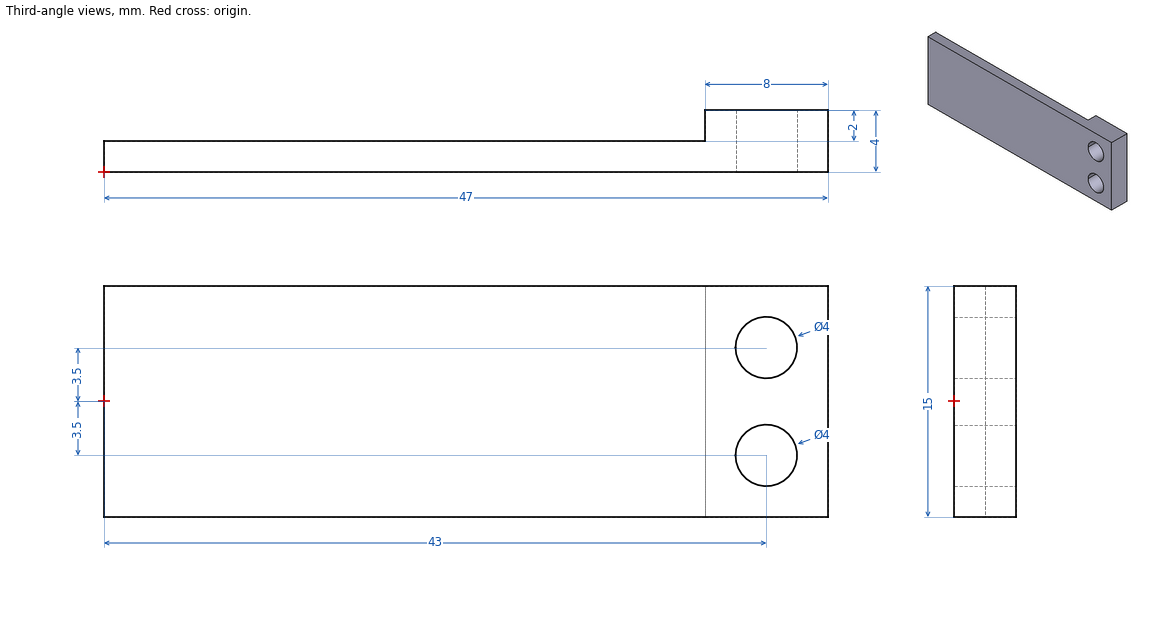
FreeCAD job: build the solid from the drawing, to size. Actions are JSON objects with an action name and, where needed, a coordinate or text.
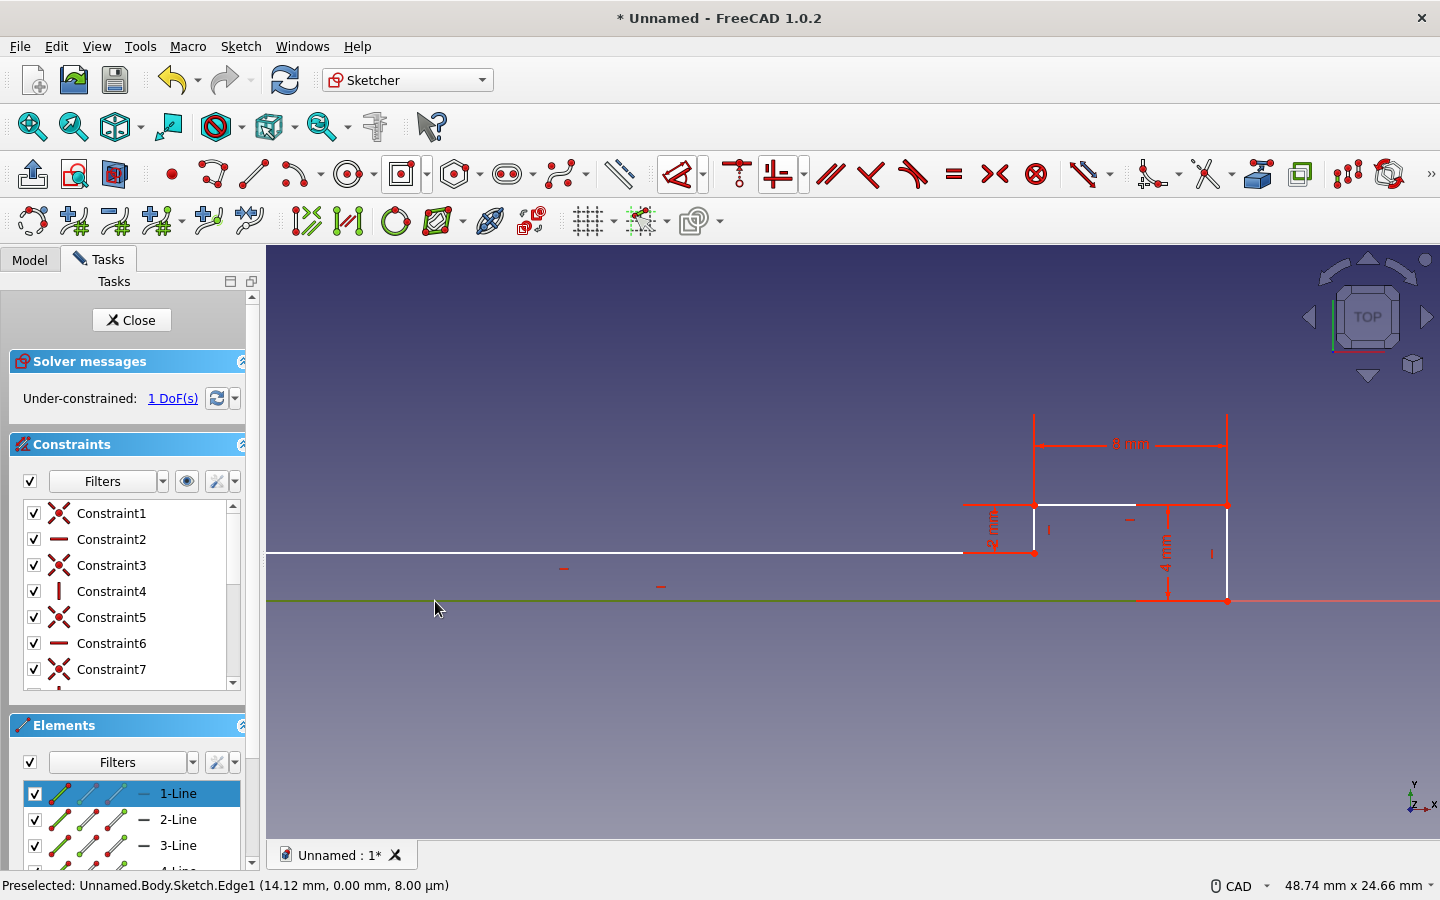
{"action": "left_click", "coordinate": [702, 174]}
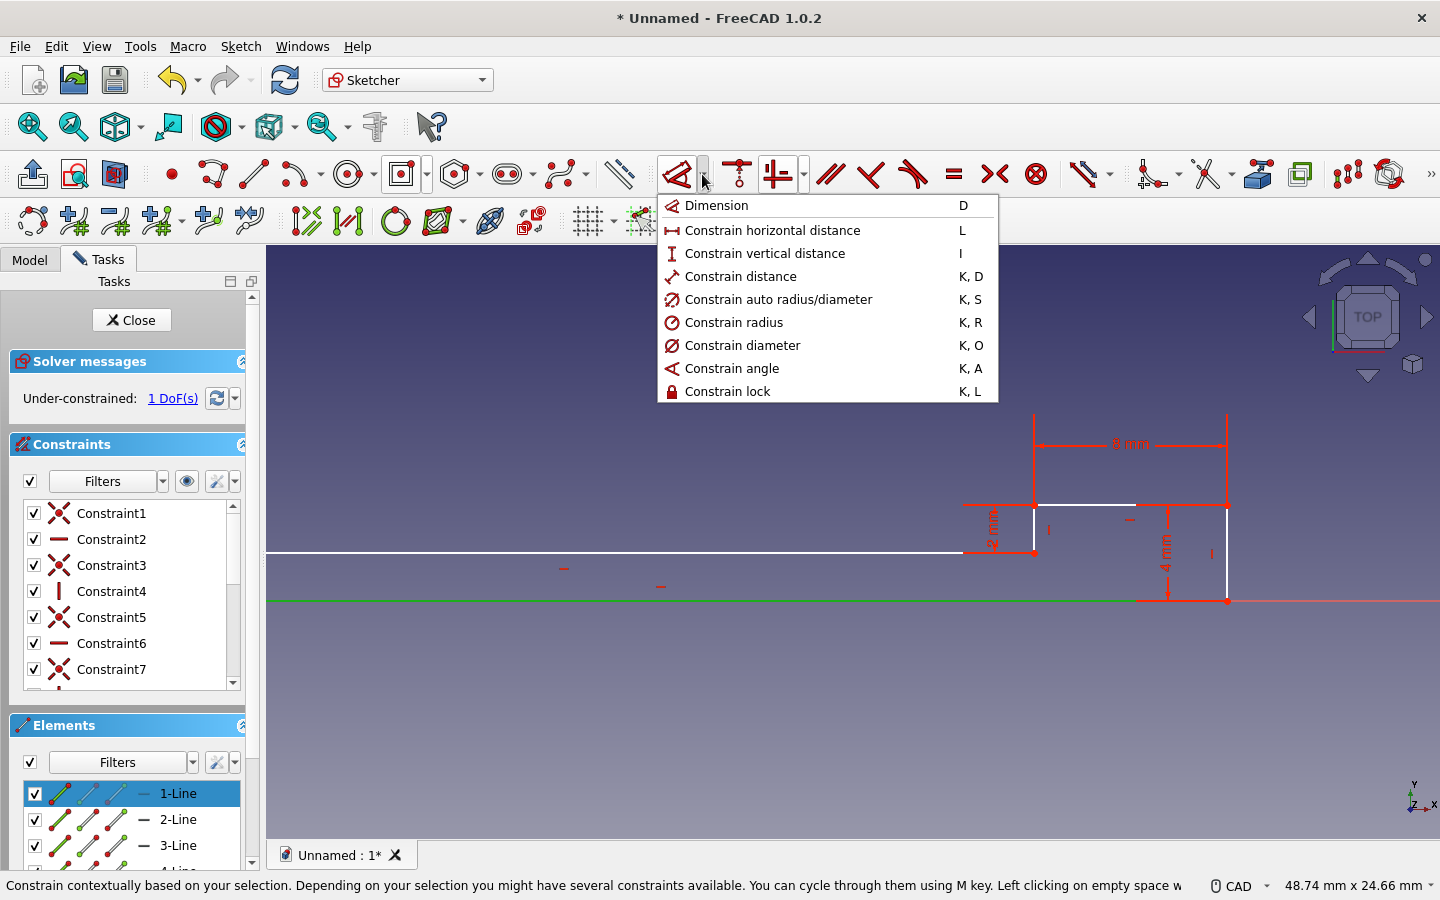
{"action": "left_click", "coordinate": [828, 230]}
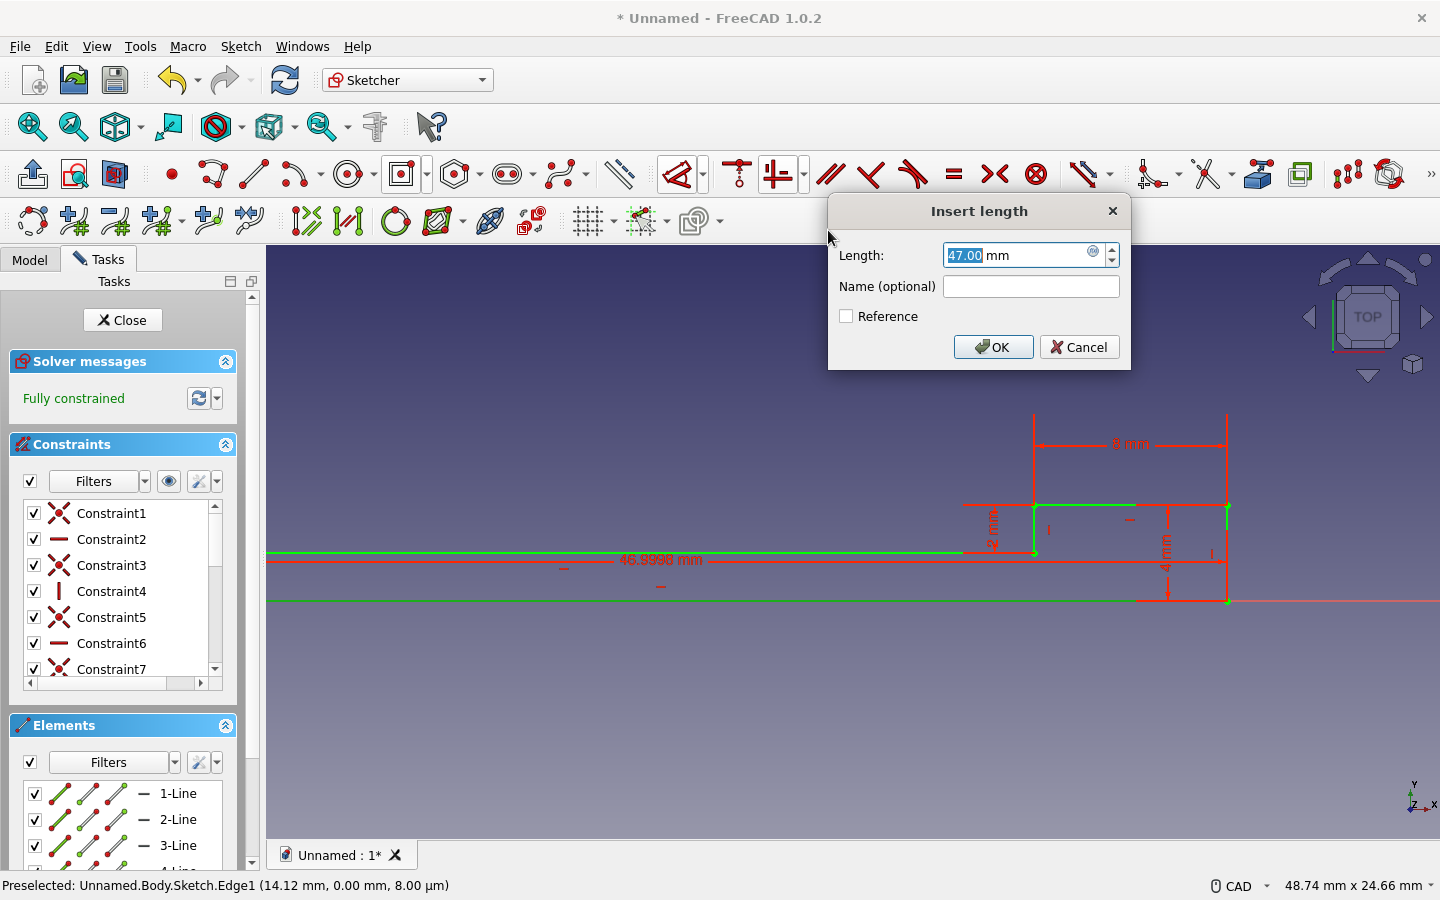
{"action": "type", "text": "47"}
{"action": "key", "text": "Return"}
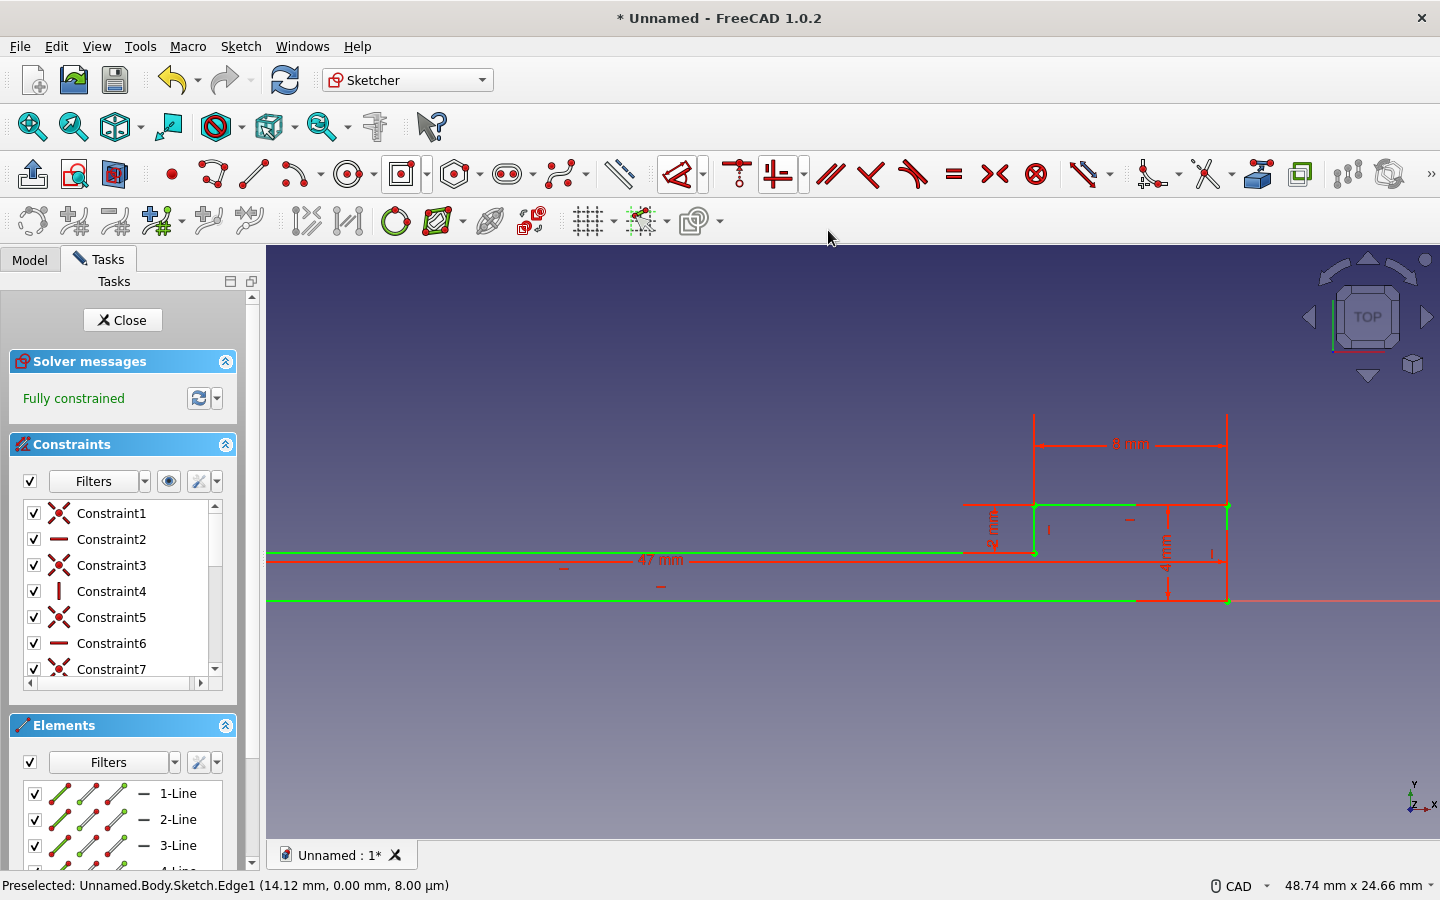
{"action": "left_click", "coordinate": [123, 320]}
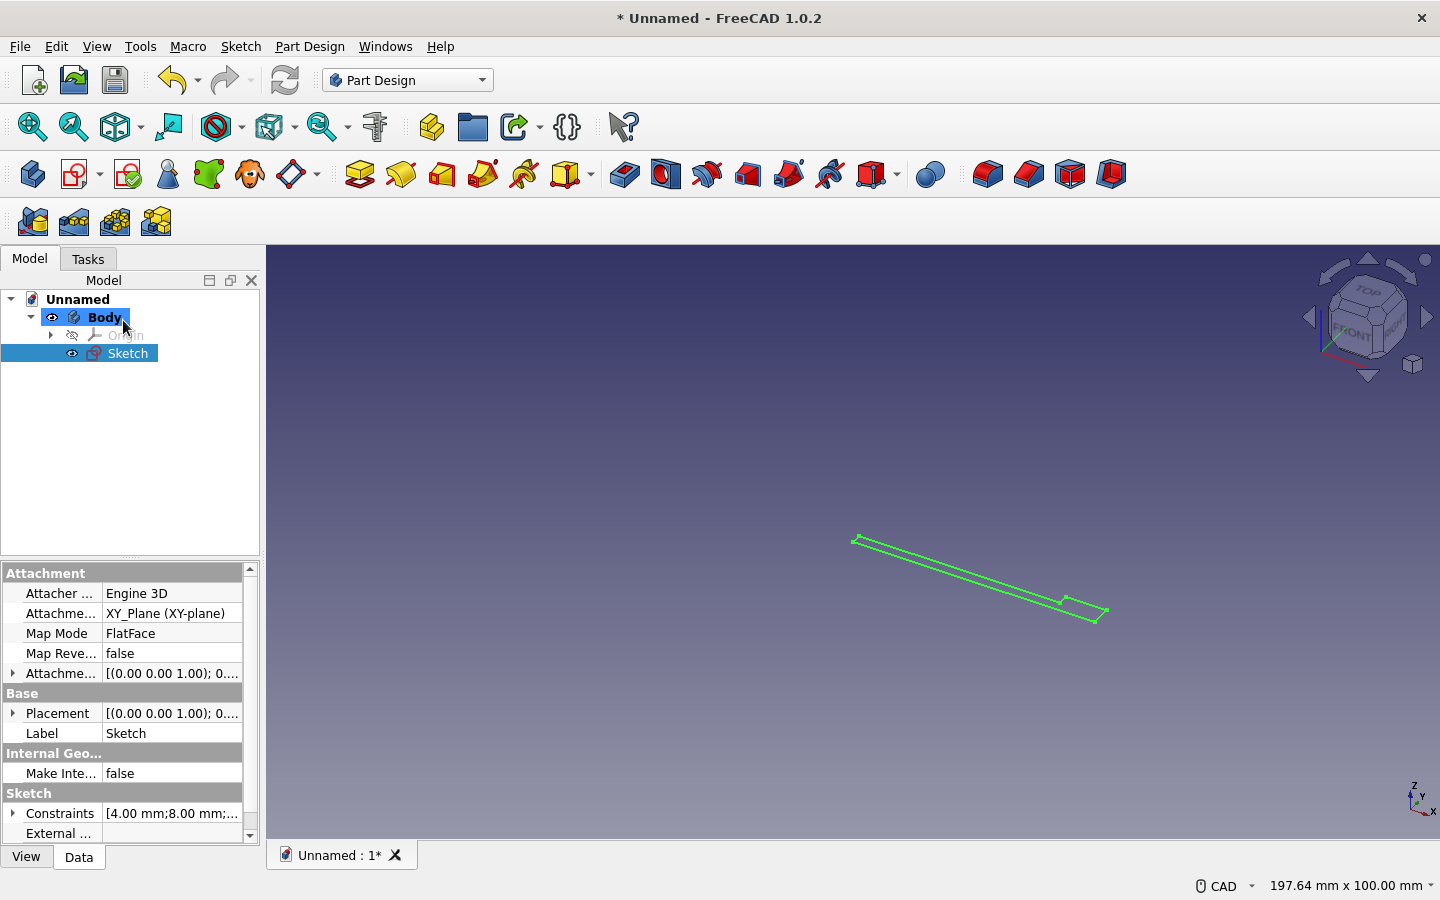
{"action": "left_click", "coordinate": [360, 174]}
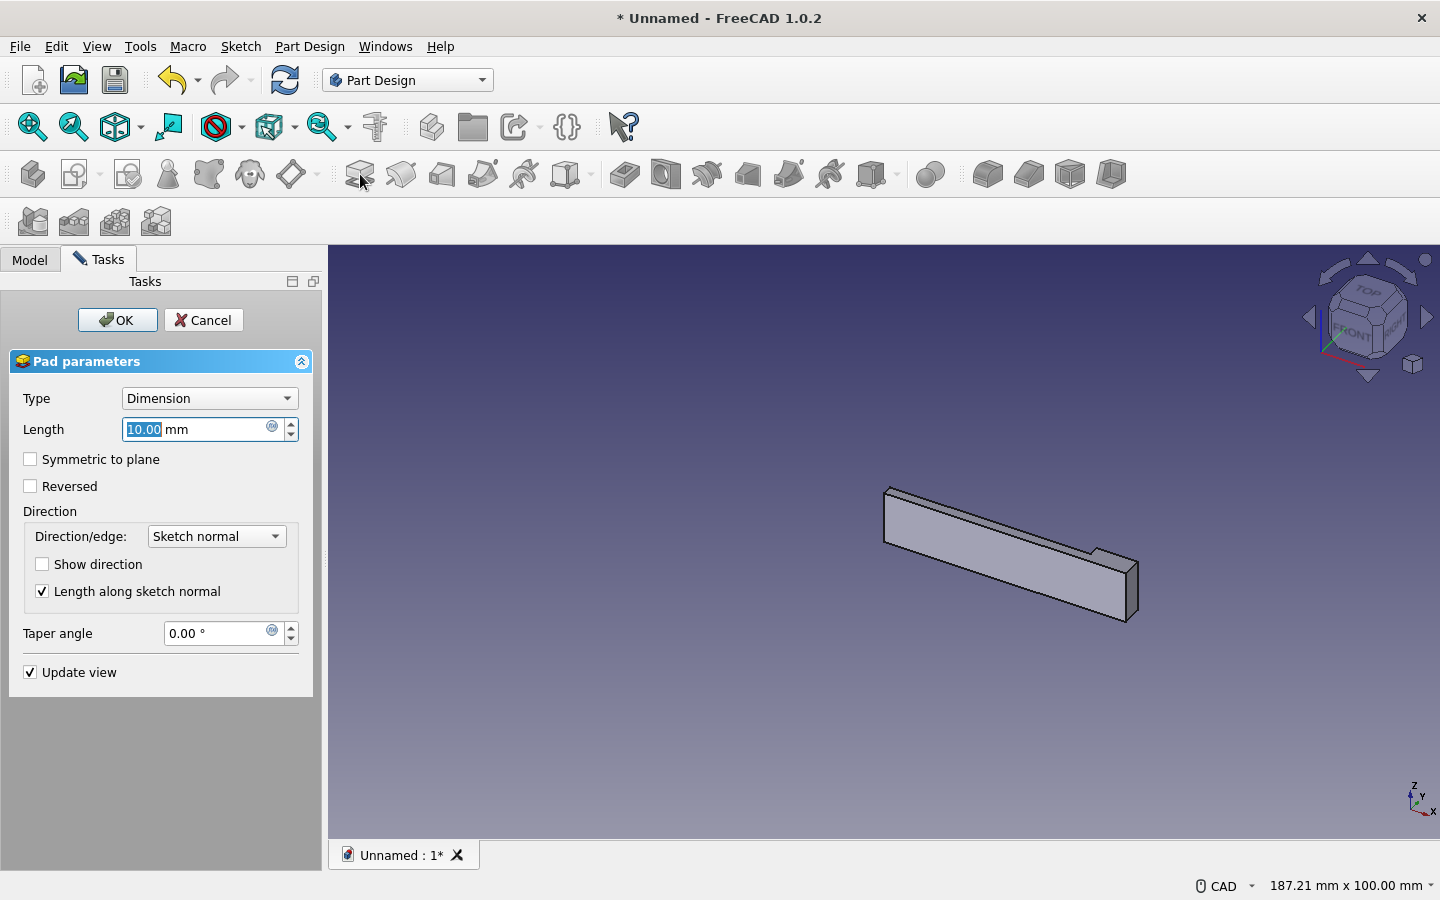
{"action": "type", "text": "15"}
{"action": "key", "text": "Tab"}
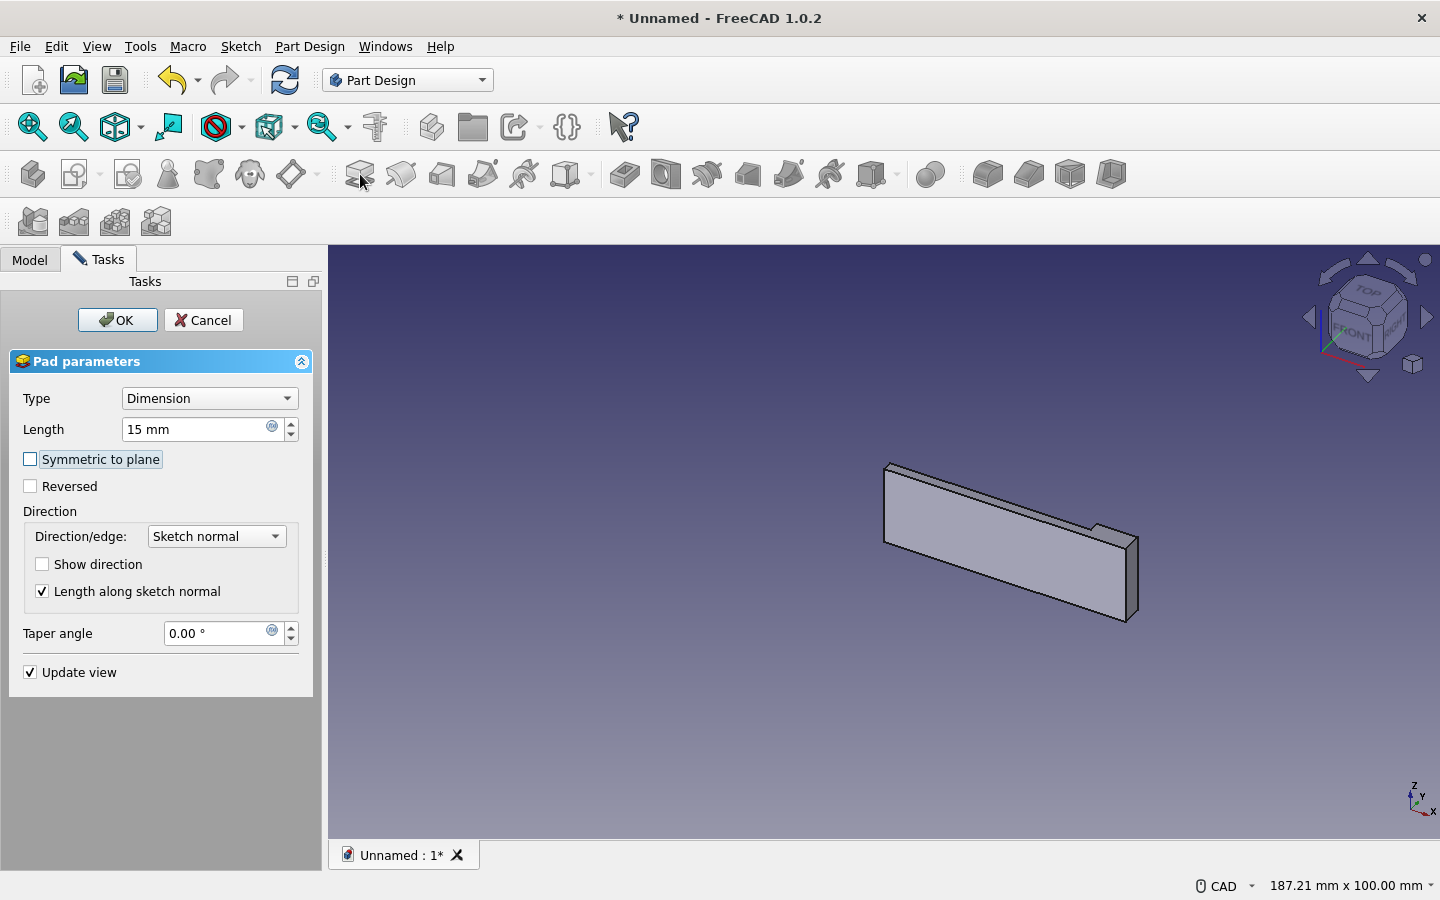
{"action": "left_click", "coordinate": [31, 459]}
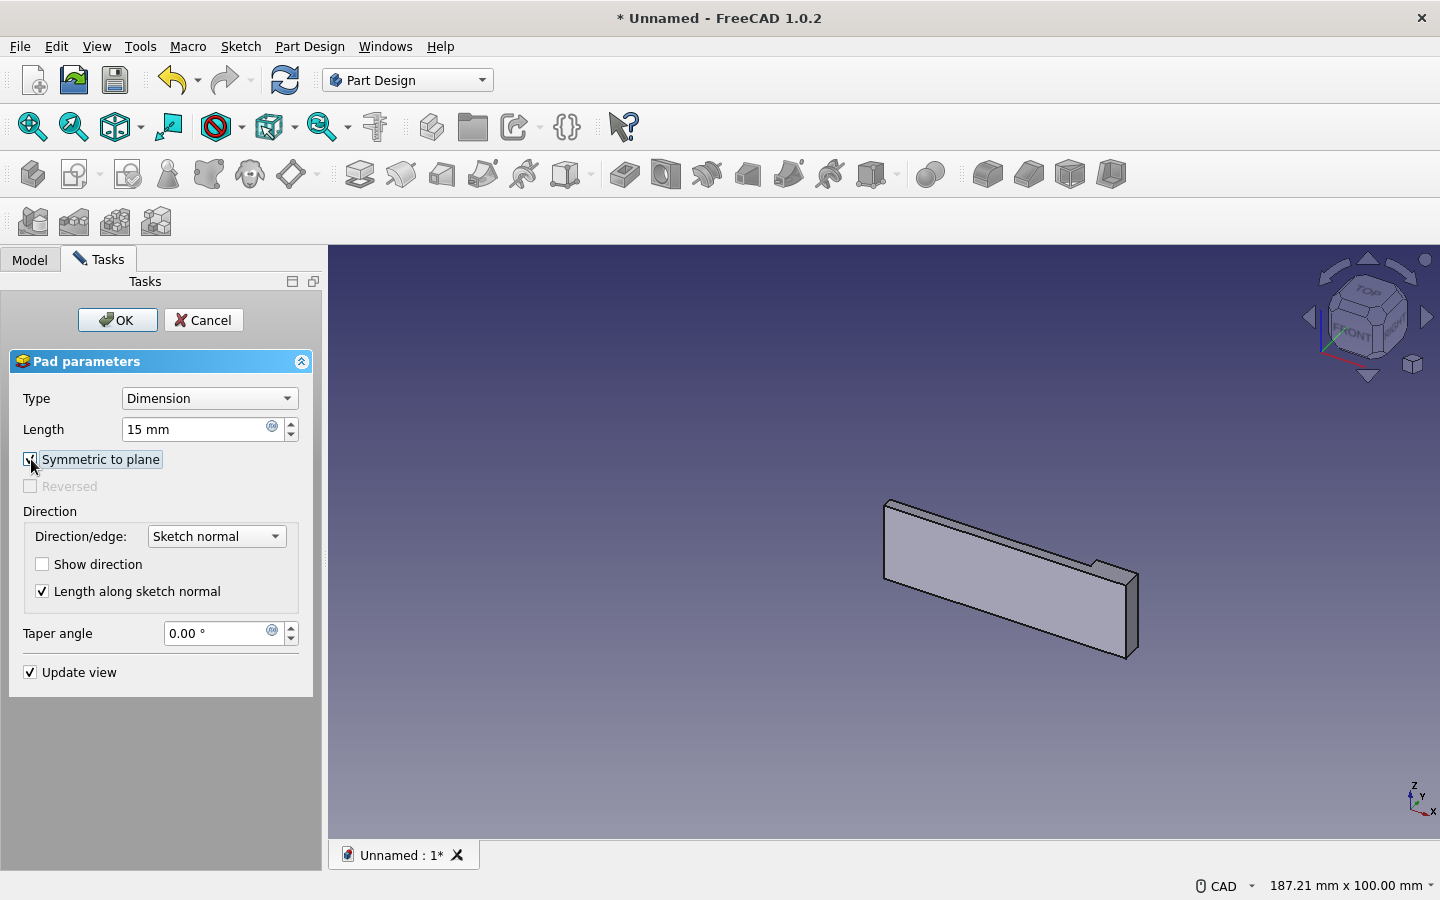
{"action": "left_click", "coordinate": [118, 320]}